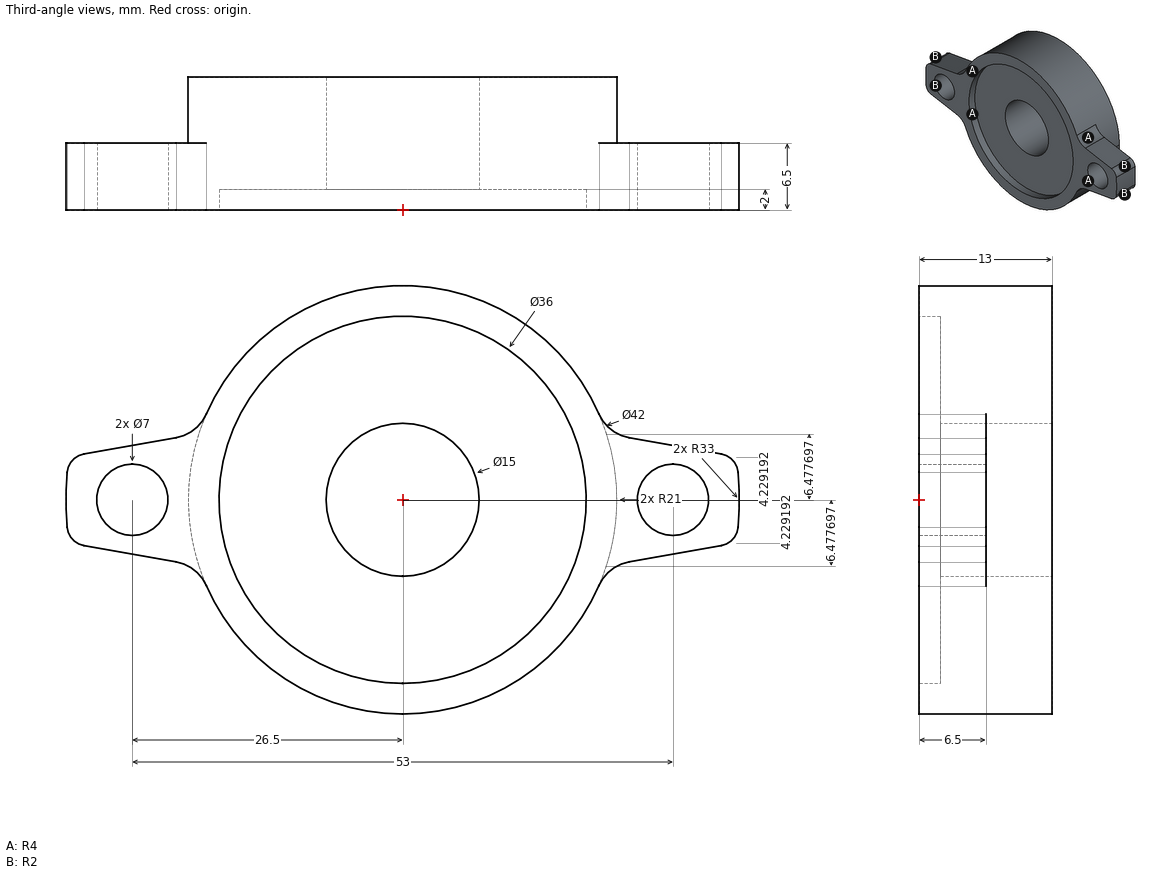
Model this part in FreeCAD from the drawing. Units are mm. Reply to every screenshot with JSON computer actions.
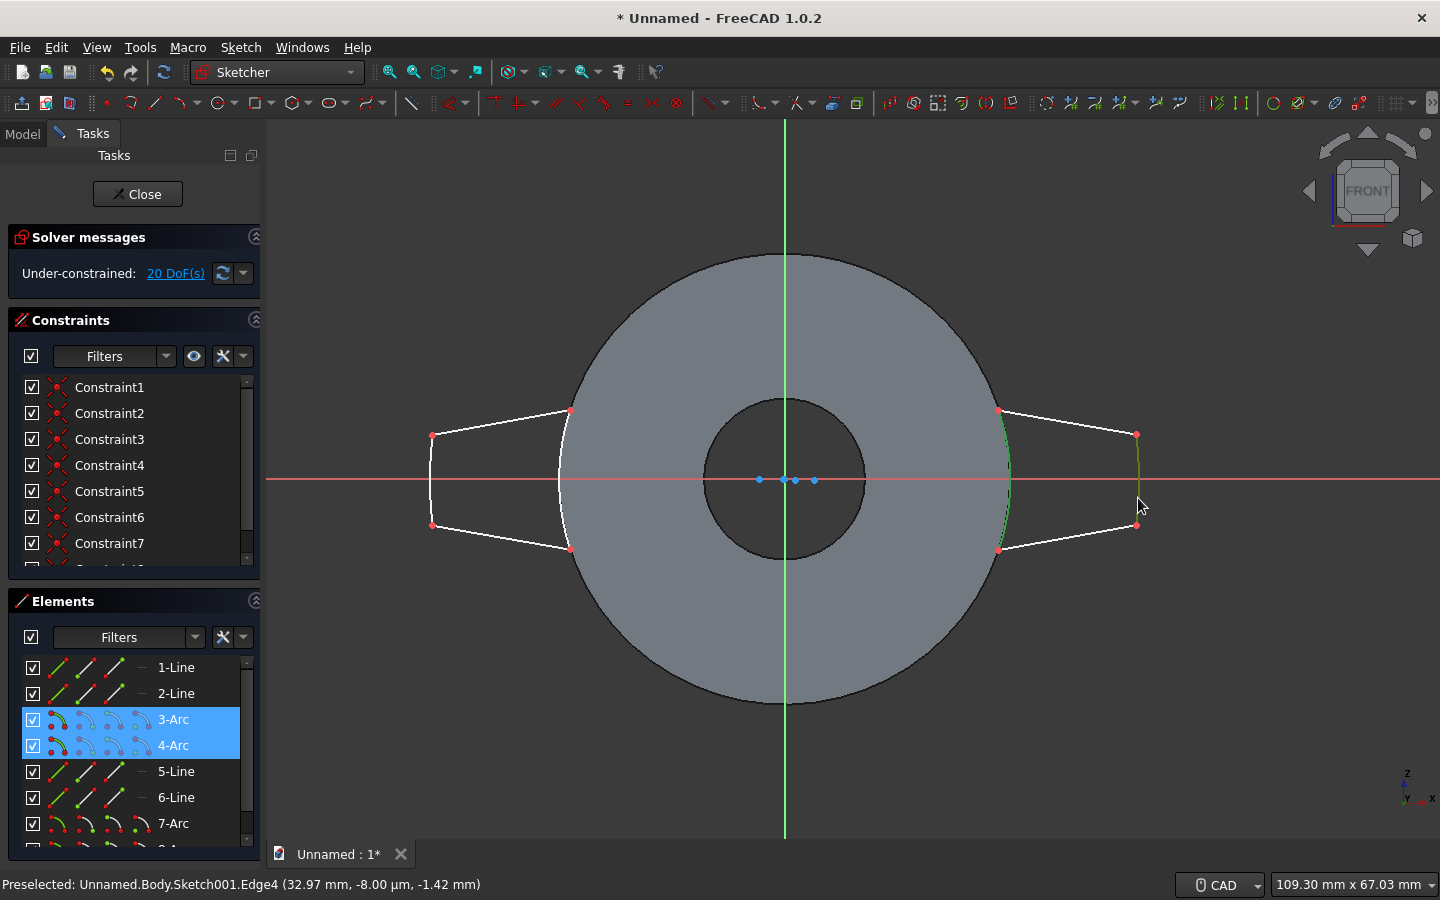
{"action": "left_click", "coordinate": [496, 104]}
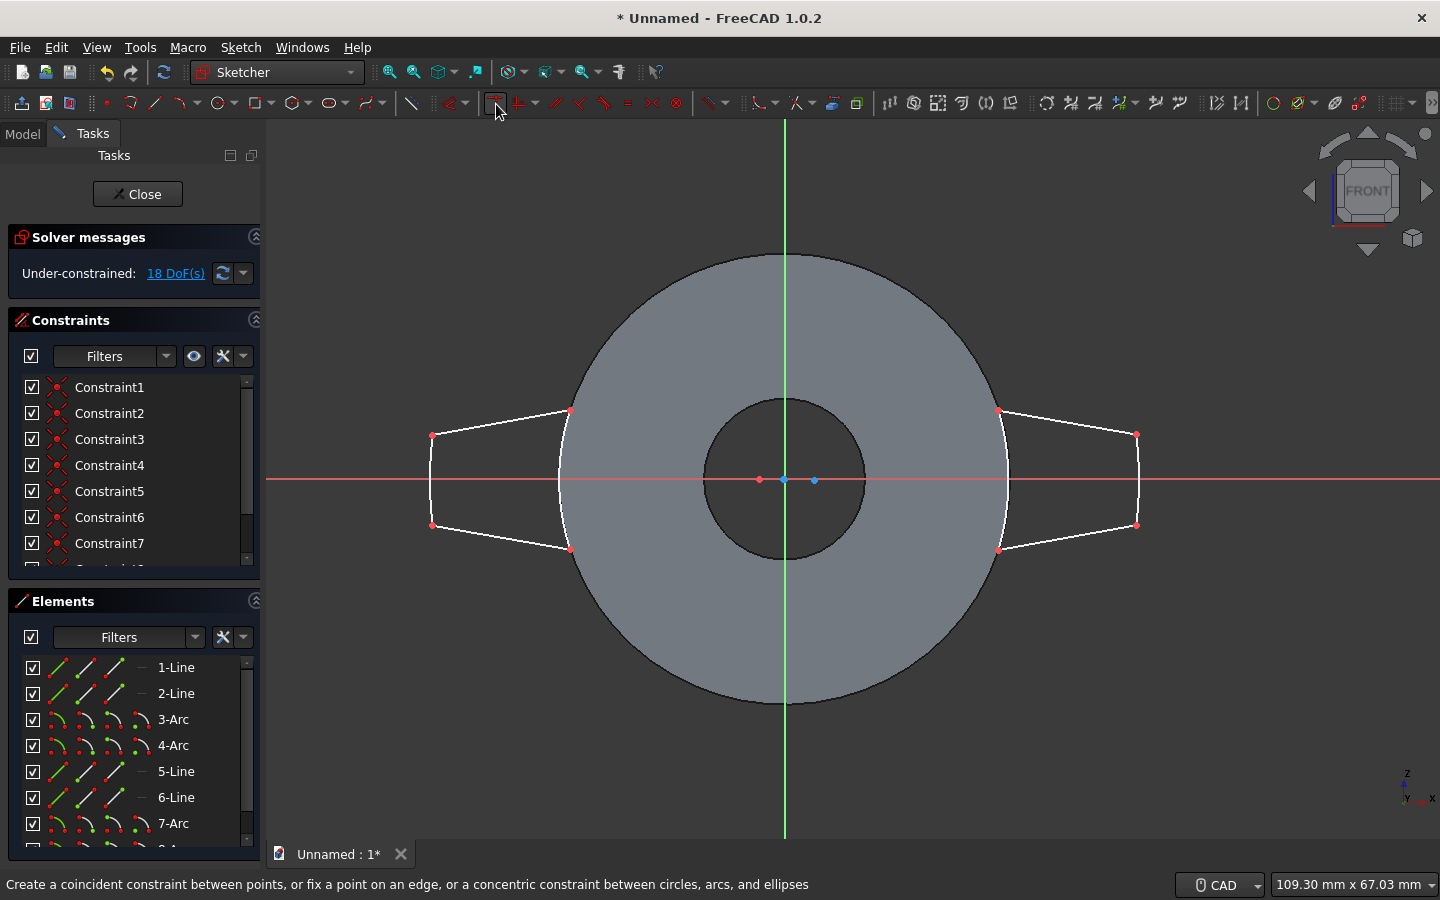
{"action": "left_click", "coordinate": [1007, 509]}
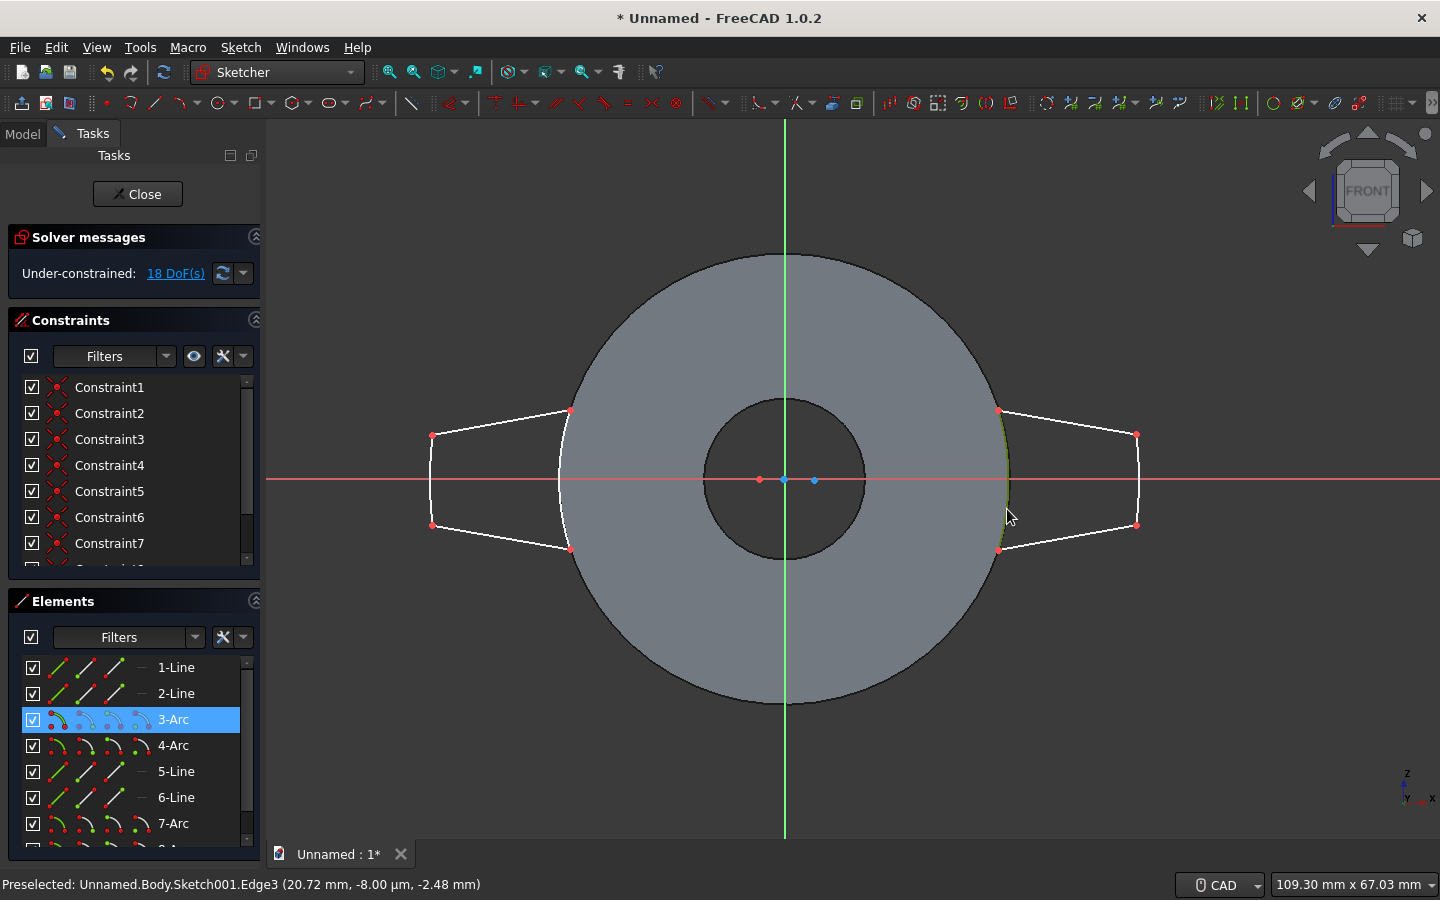
{"action": "left_click", "coordinate": [561, 452]}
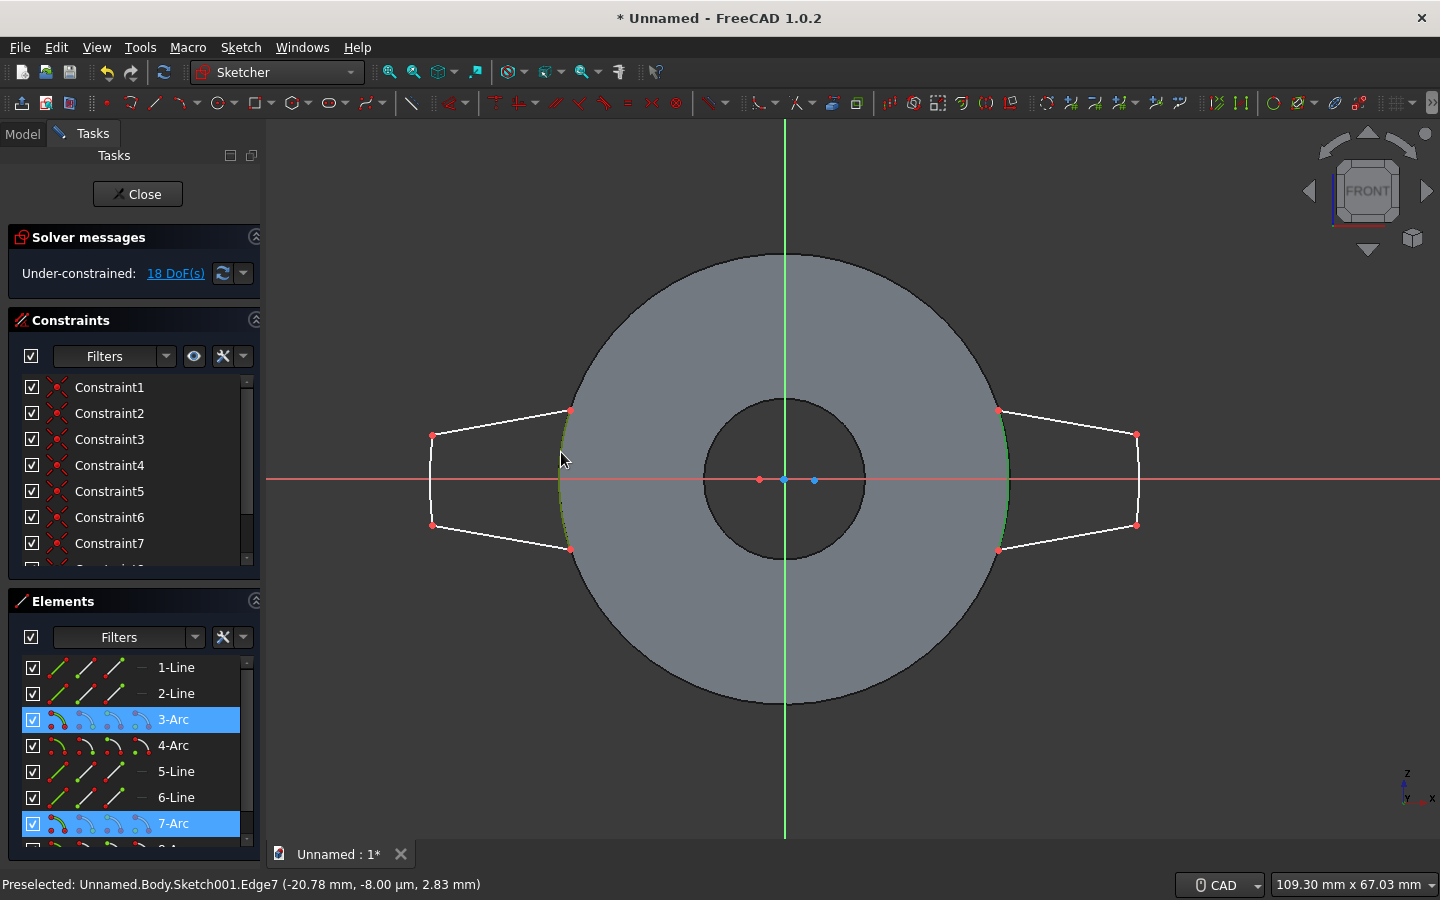
{"action": "left_click", "coordinate": [496, 104]}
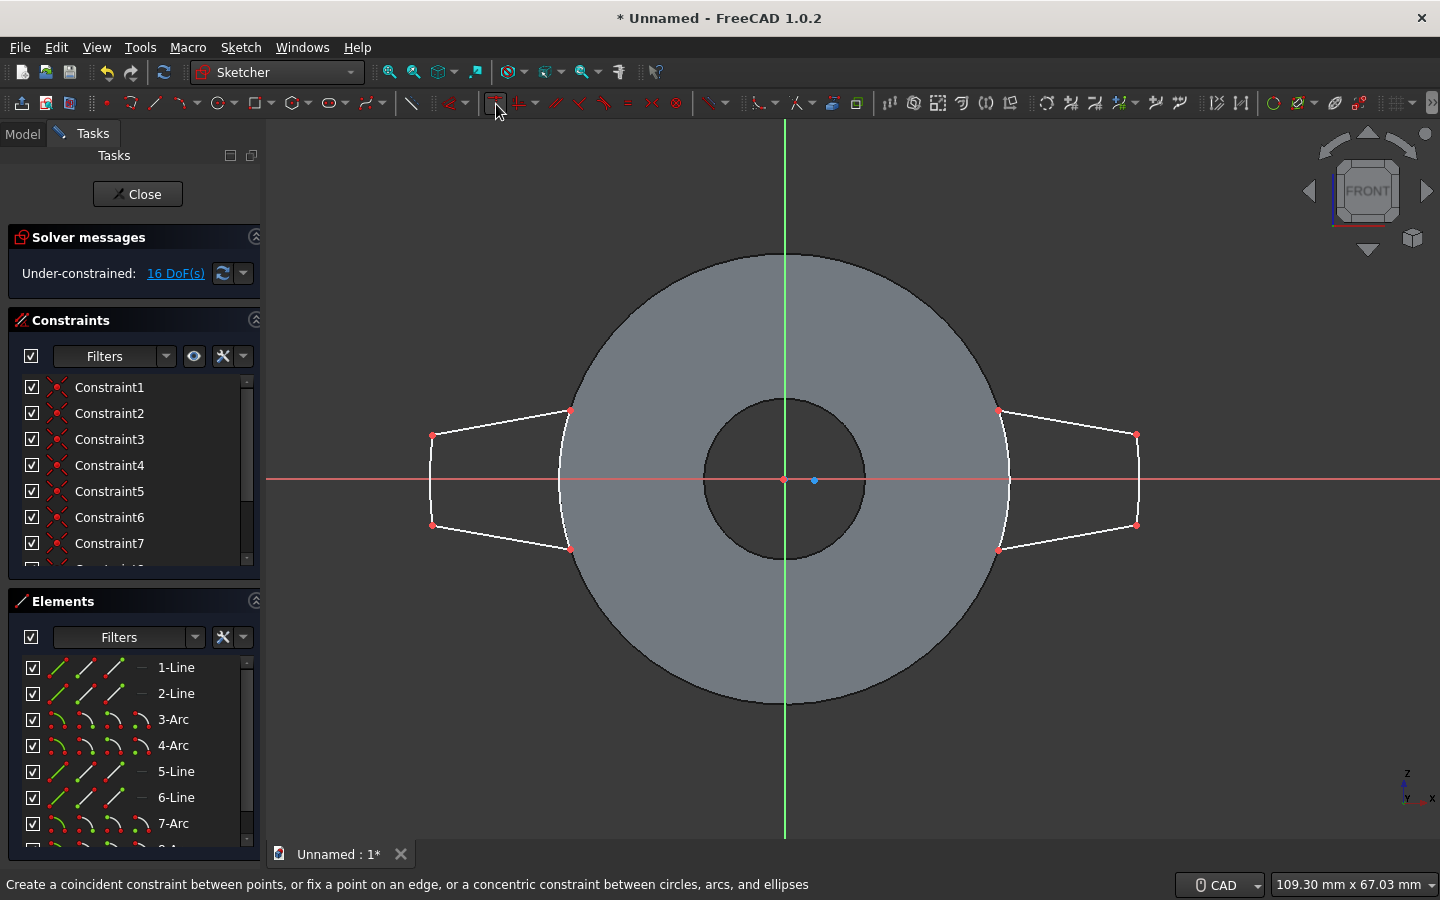
{"action": "left_click", "coordinate": [1008, 509]}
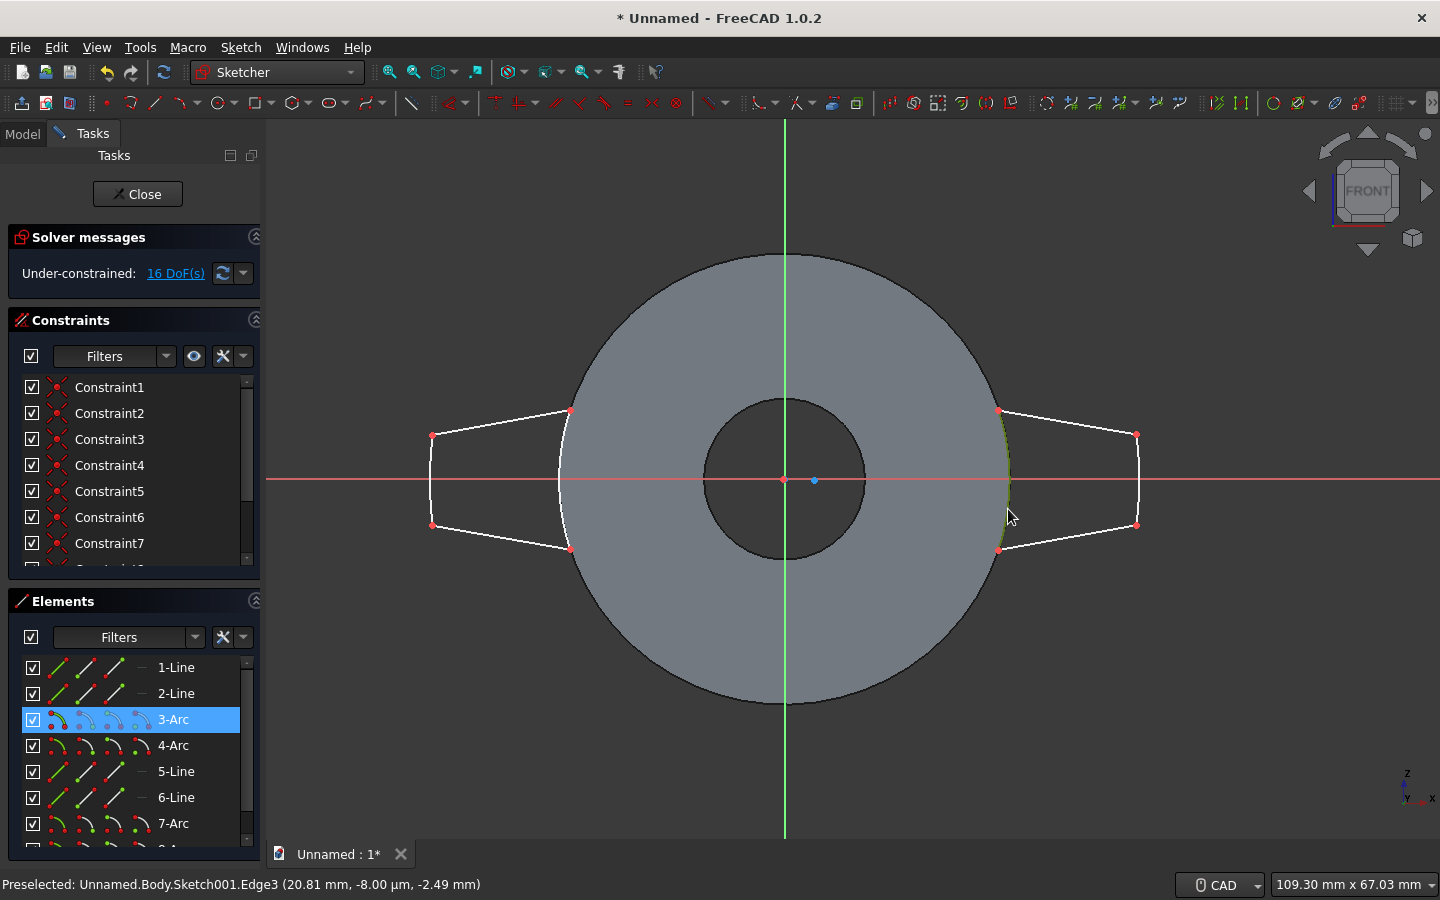
{"action": "left_click", "coordinate": [430, 462]}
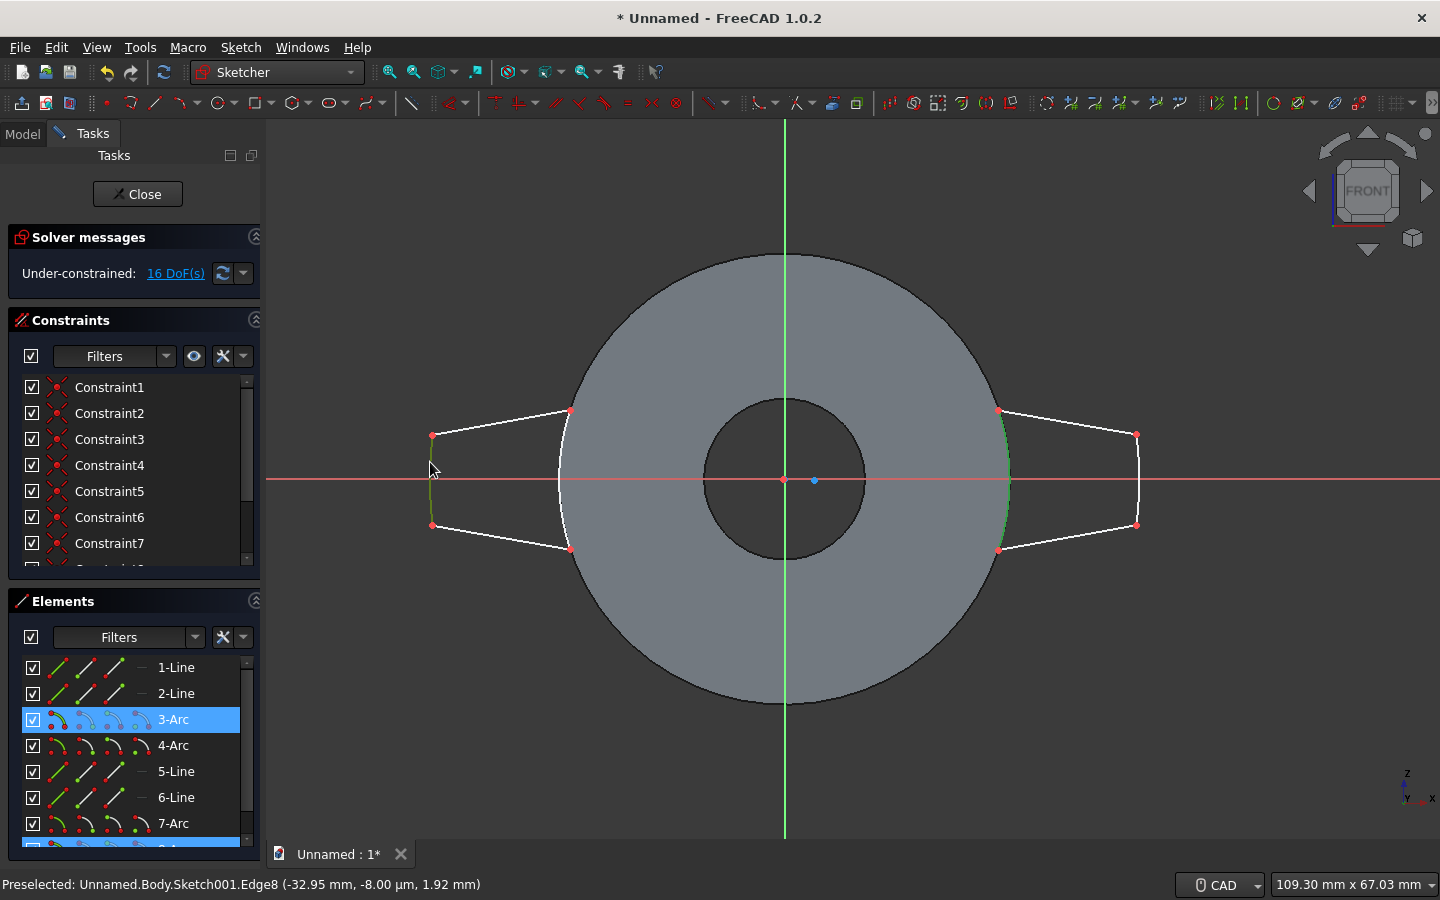
{"action": "left_click", "coordinate": [496, 104]}